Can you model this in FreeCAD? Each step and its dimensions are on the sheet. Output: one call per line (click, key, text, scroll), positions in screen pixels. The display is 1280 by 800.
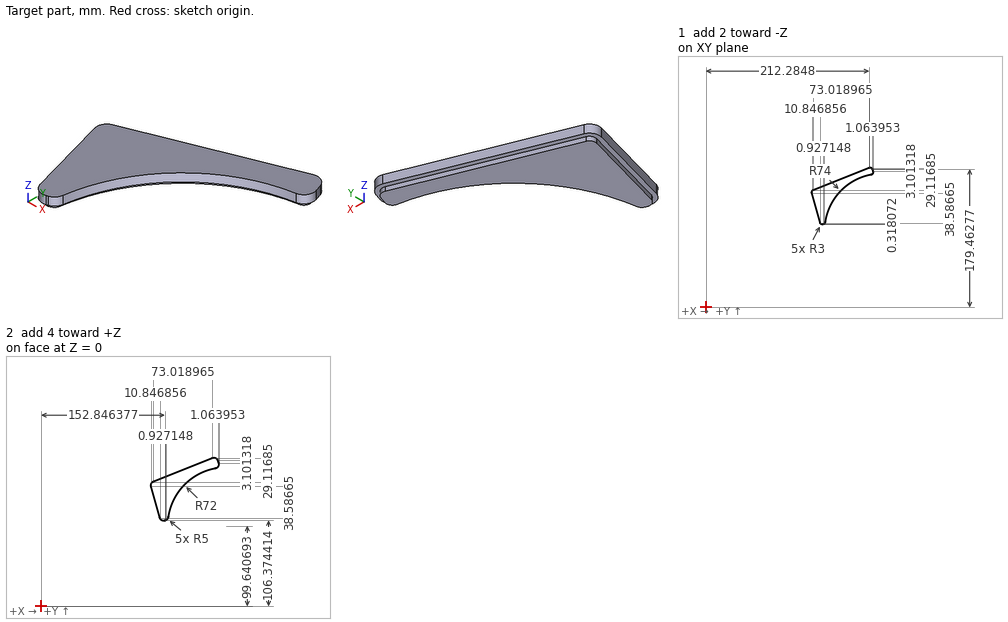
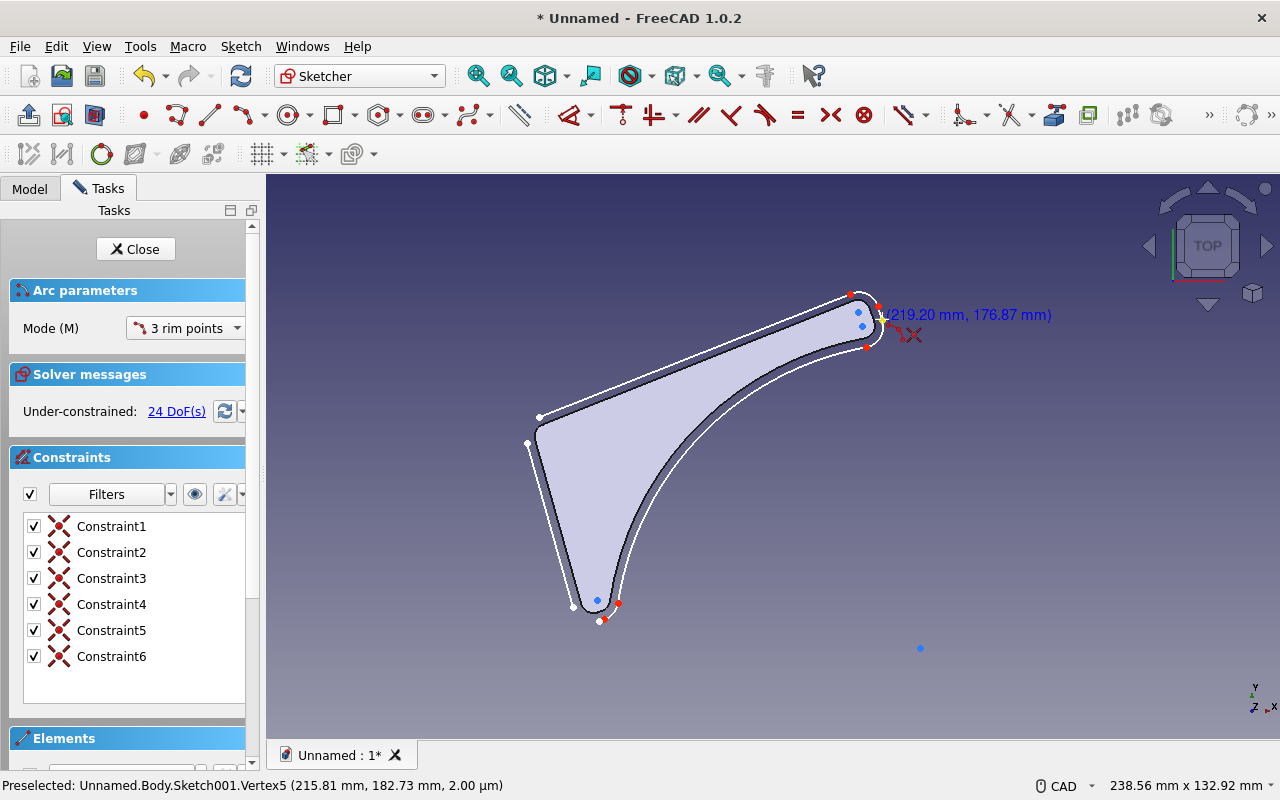
click(539, 417)
click(527, 443)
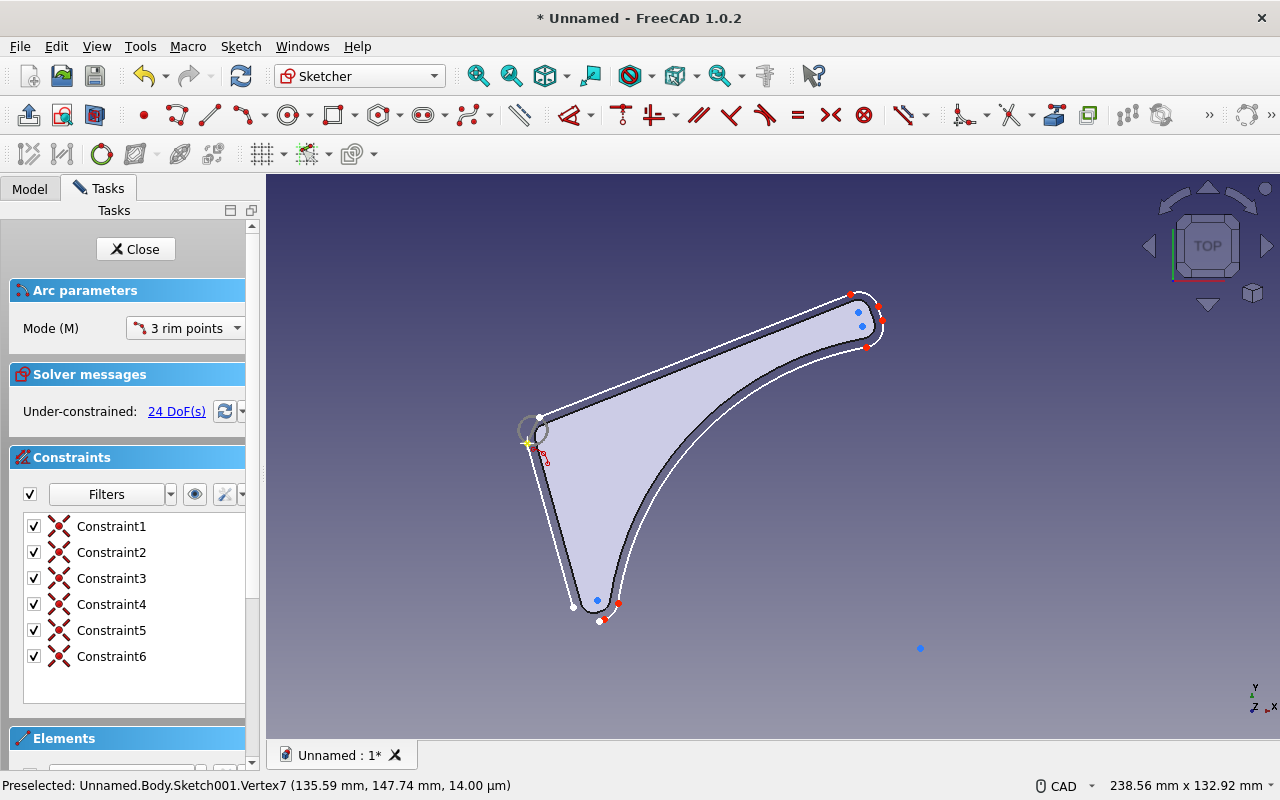
scroll(528, 427, up, 6)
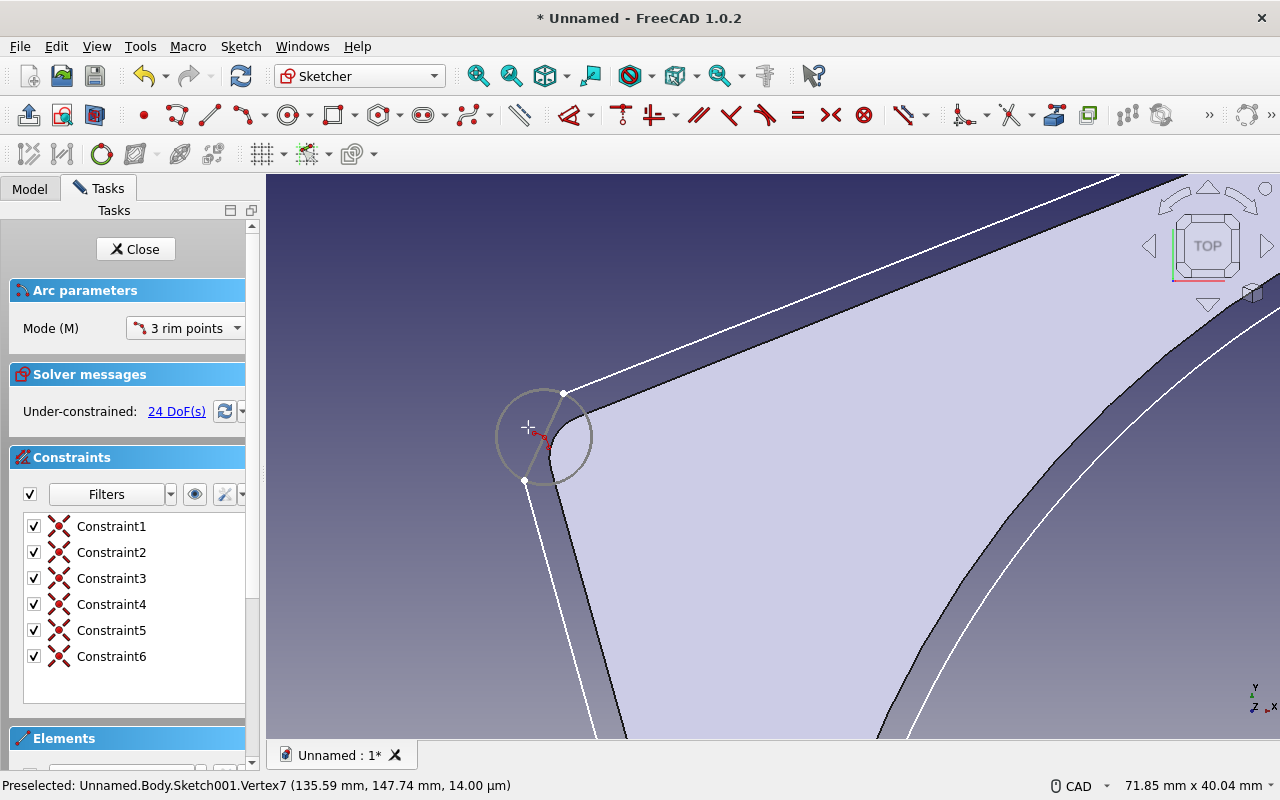
click(528, 426)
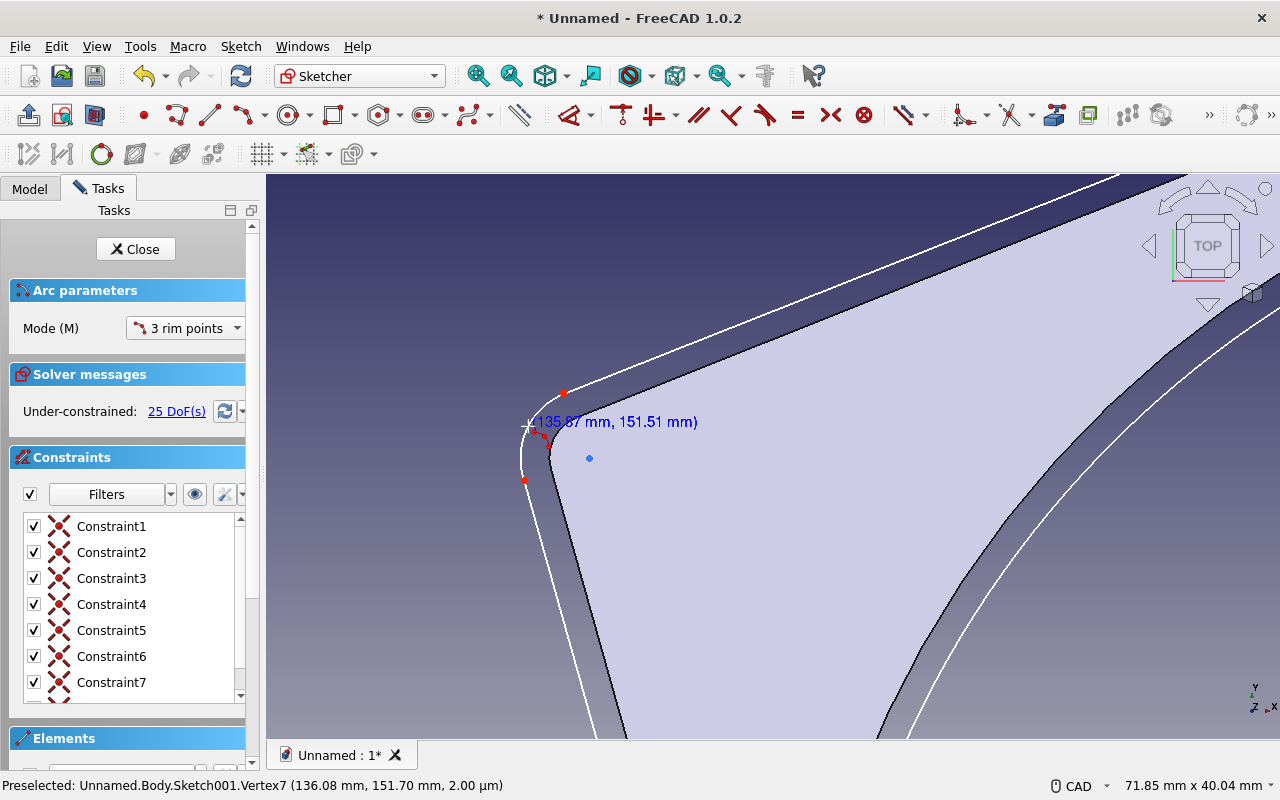
scroll(528, 427, down, 6)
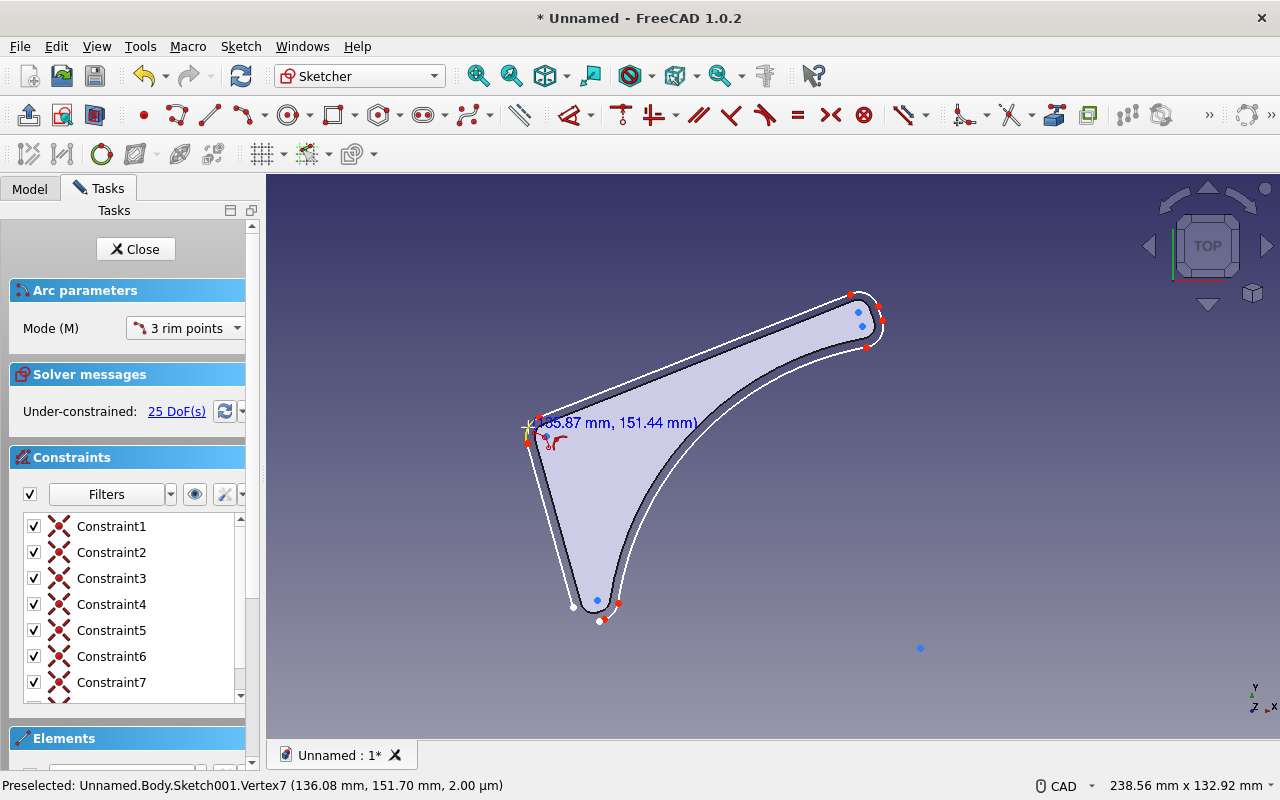
click(573, 607)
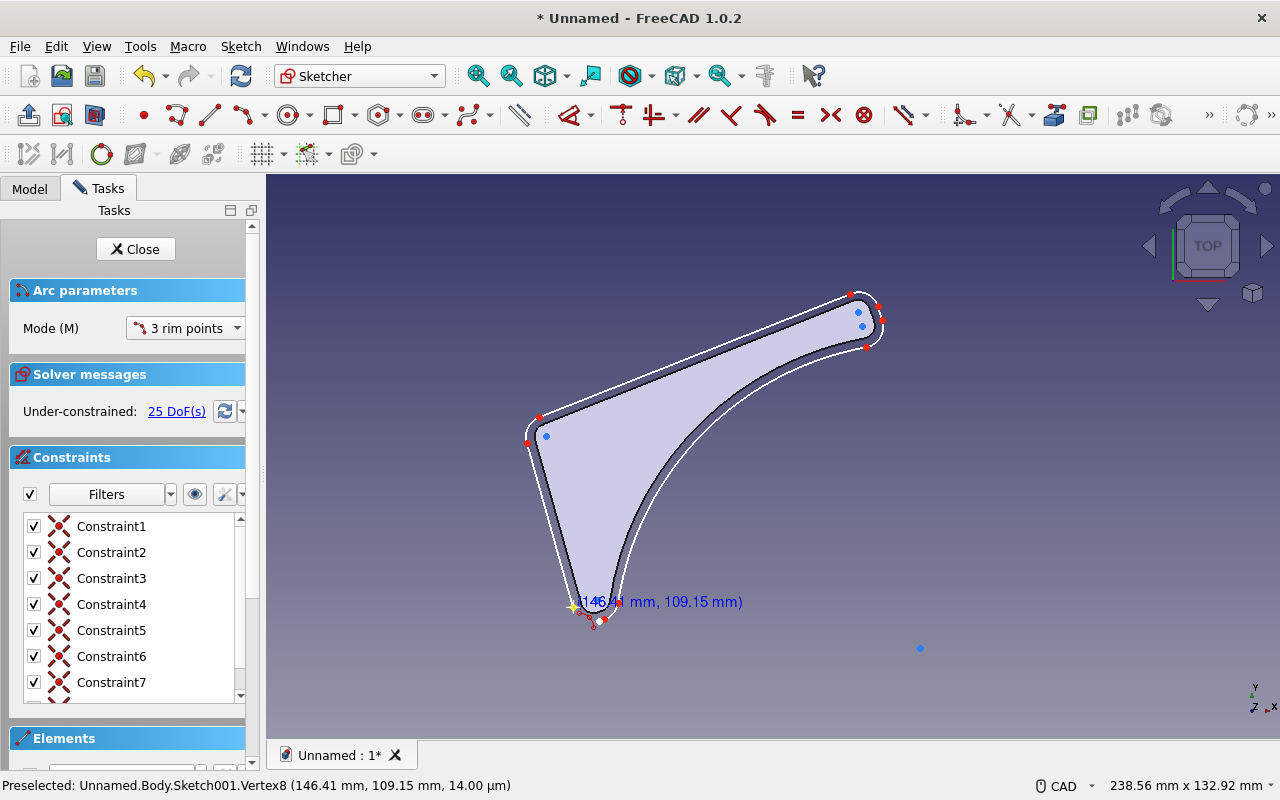
scroll(600, 621, up, 11)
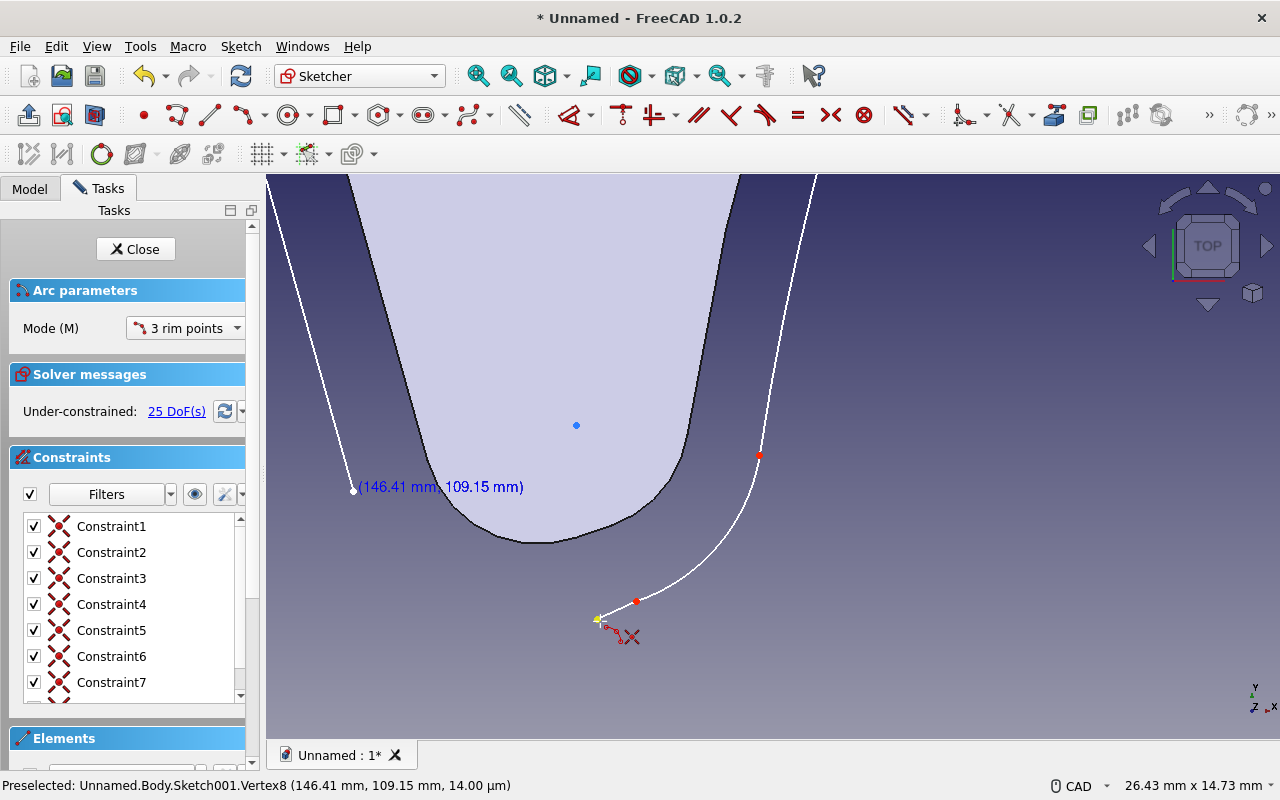
click(597, 619)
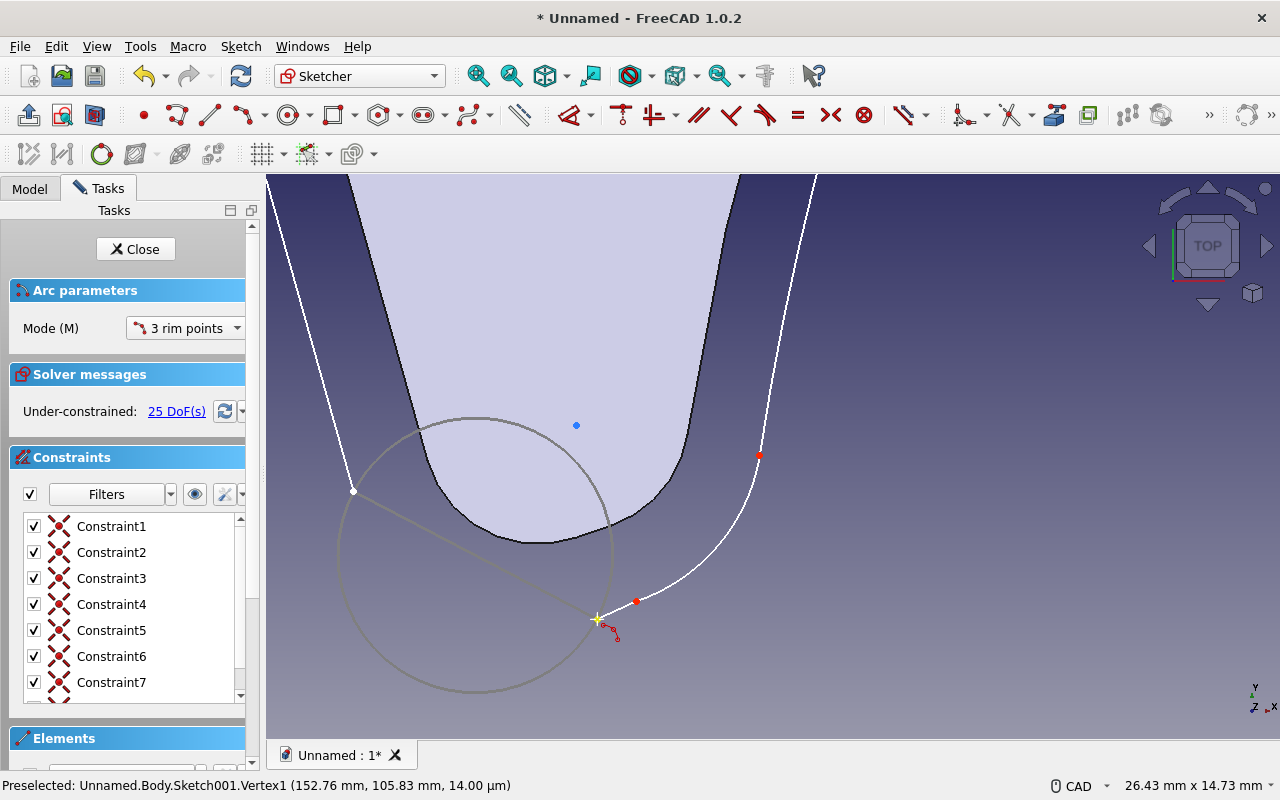
scroll(600, 622, down, 11)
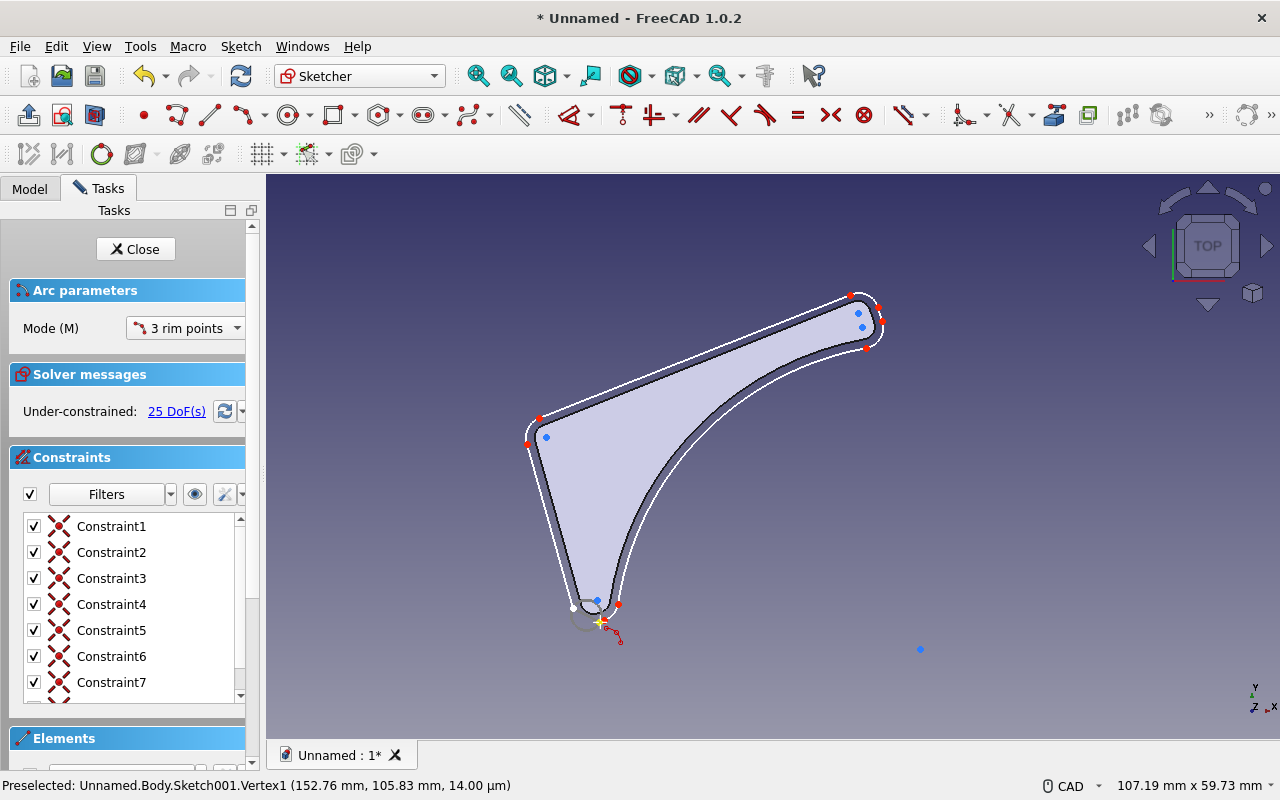
scroll(584, 620, up, 5)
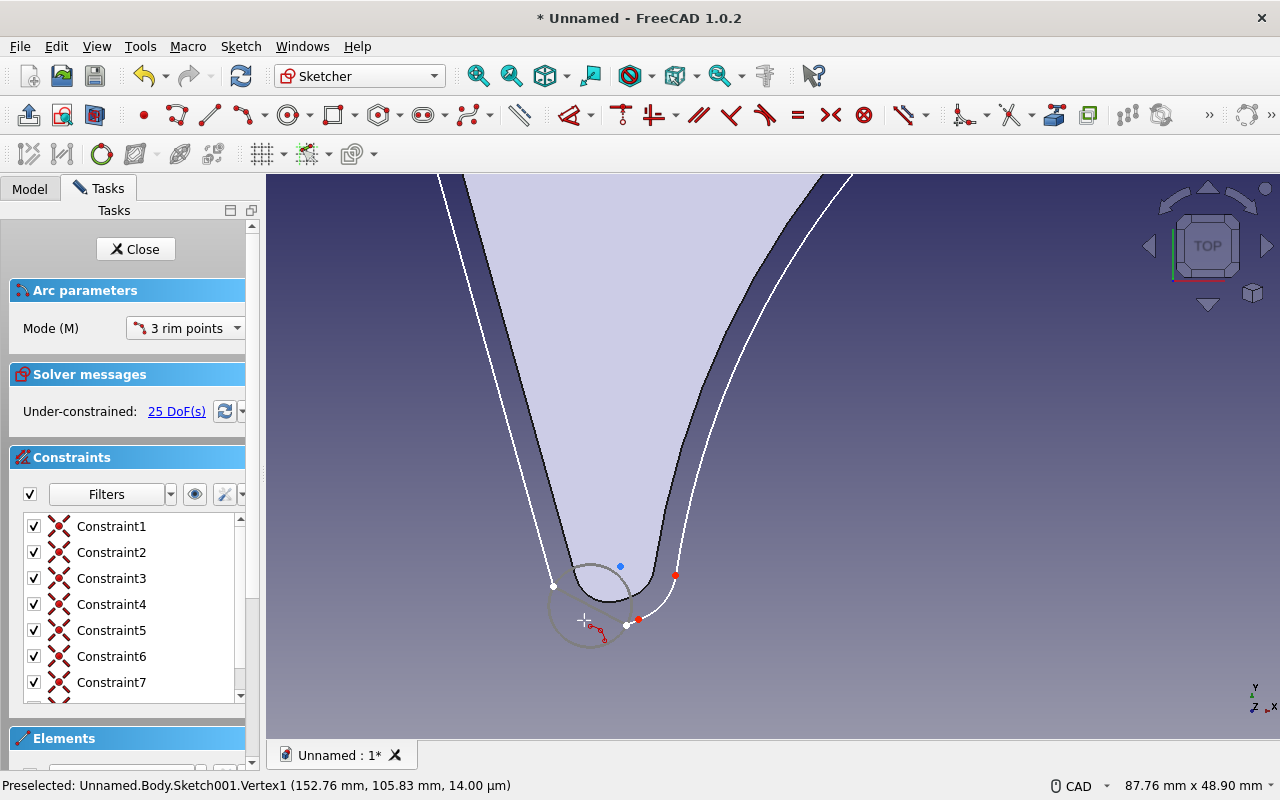
click(582, 619)
key(Escape)